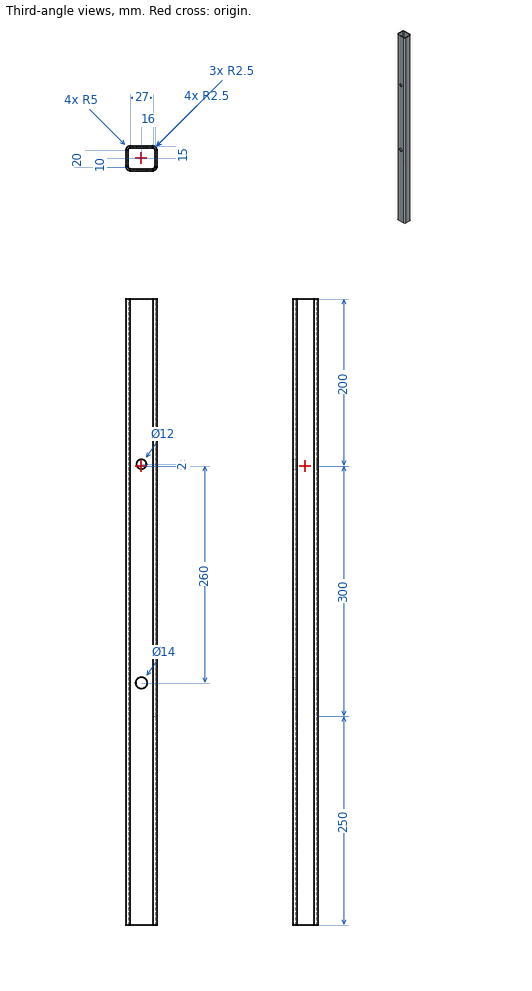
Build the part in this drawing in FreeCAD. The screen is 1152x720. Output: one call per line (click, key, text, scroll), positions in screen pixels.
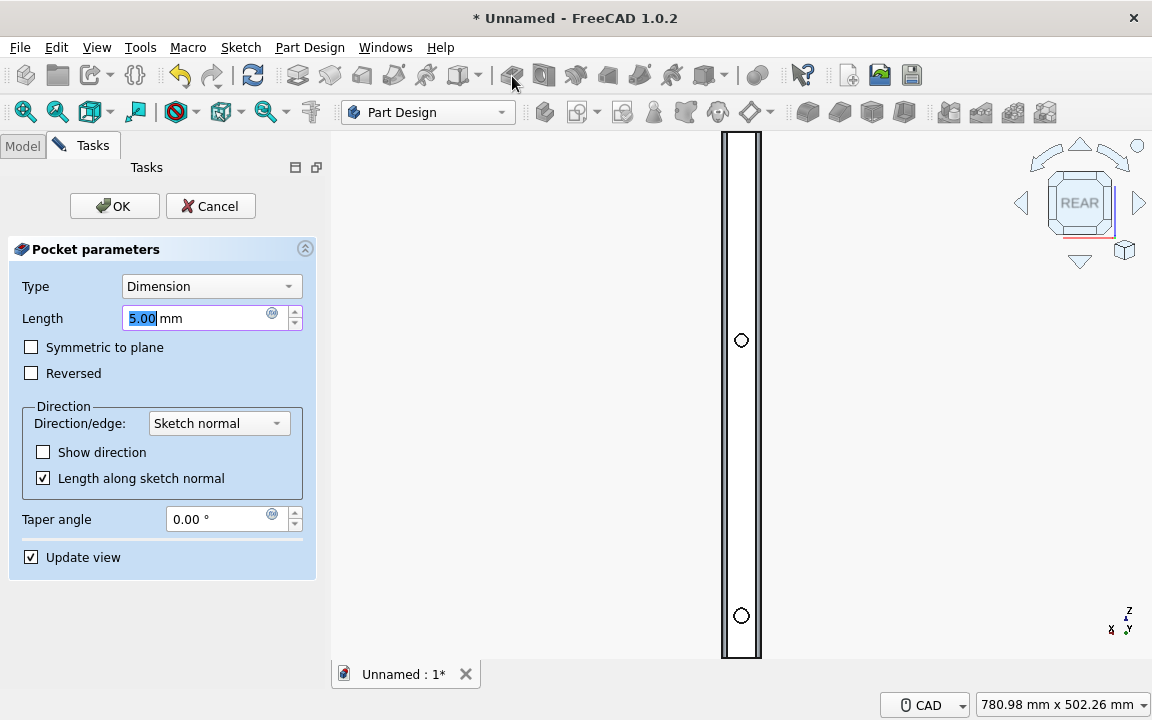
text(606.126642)
key(Tab)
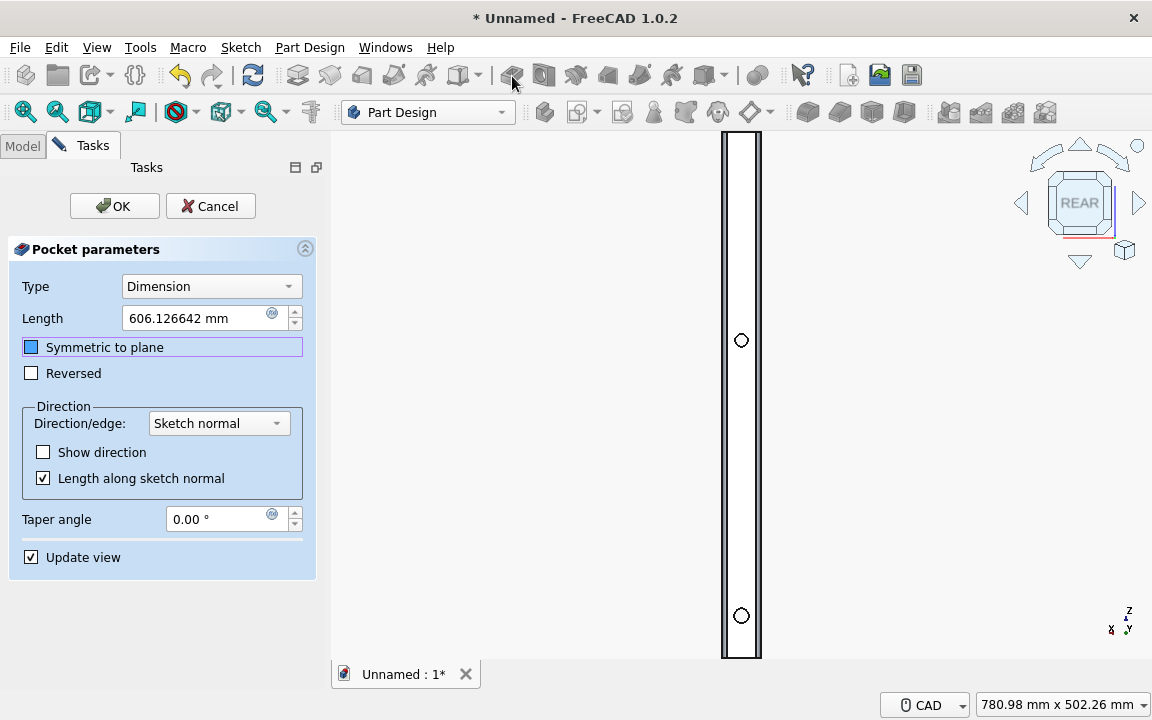
click(30, 347)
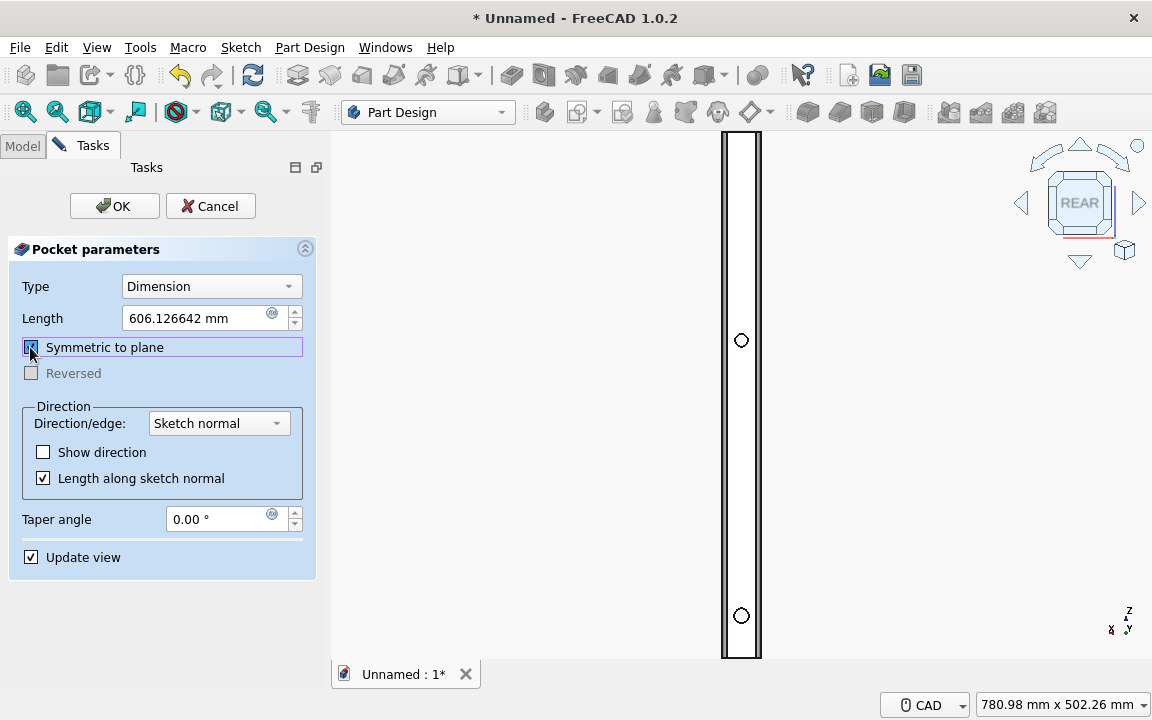
click(115, 206)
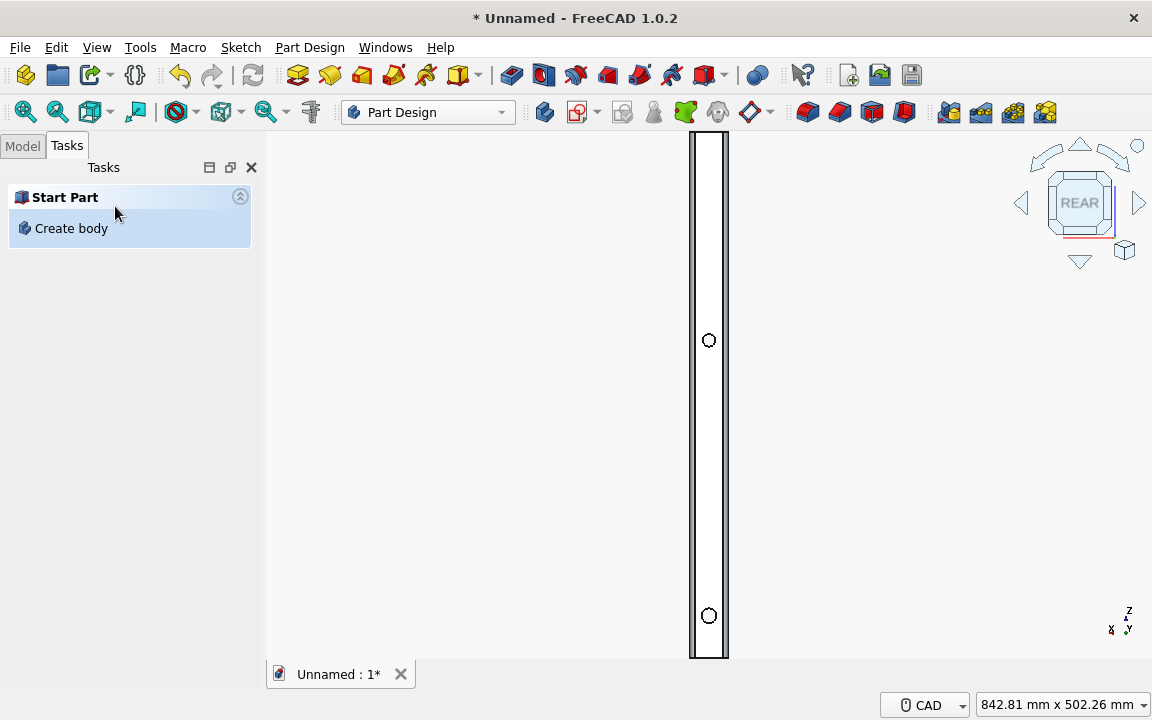
click(23, 145)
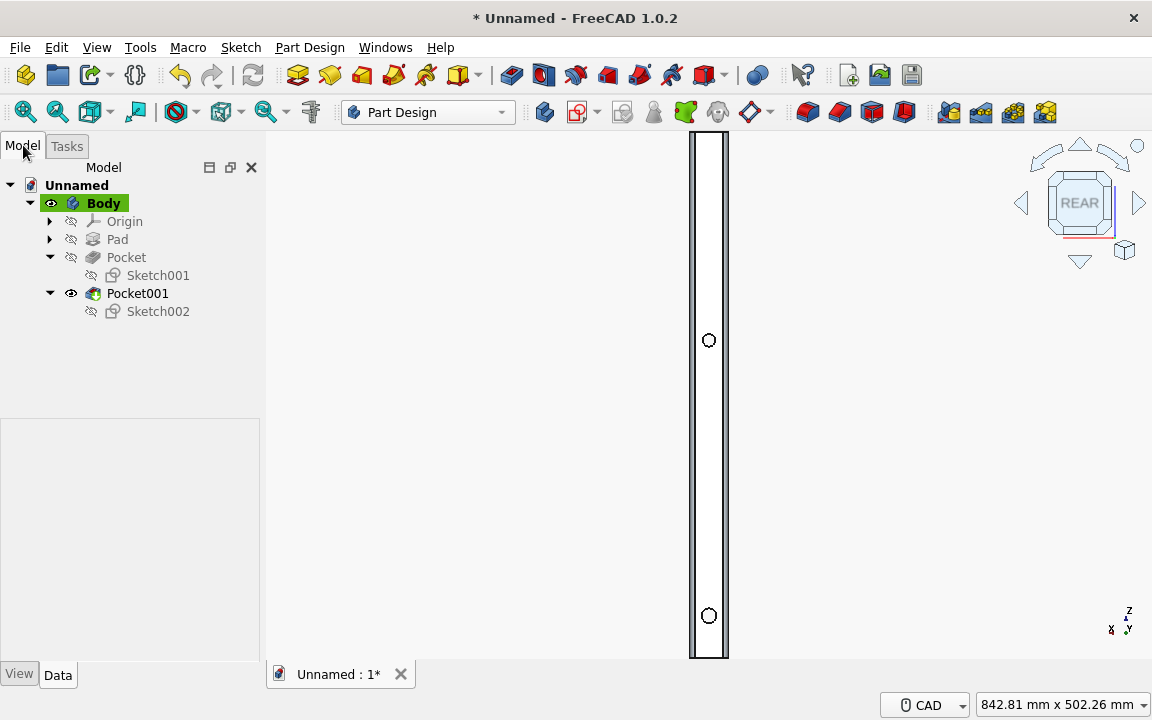
click(50, 221)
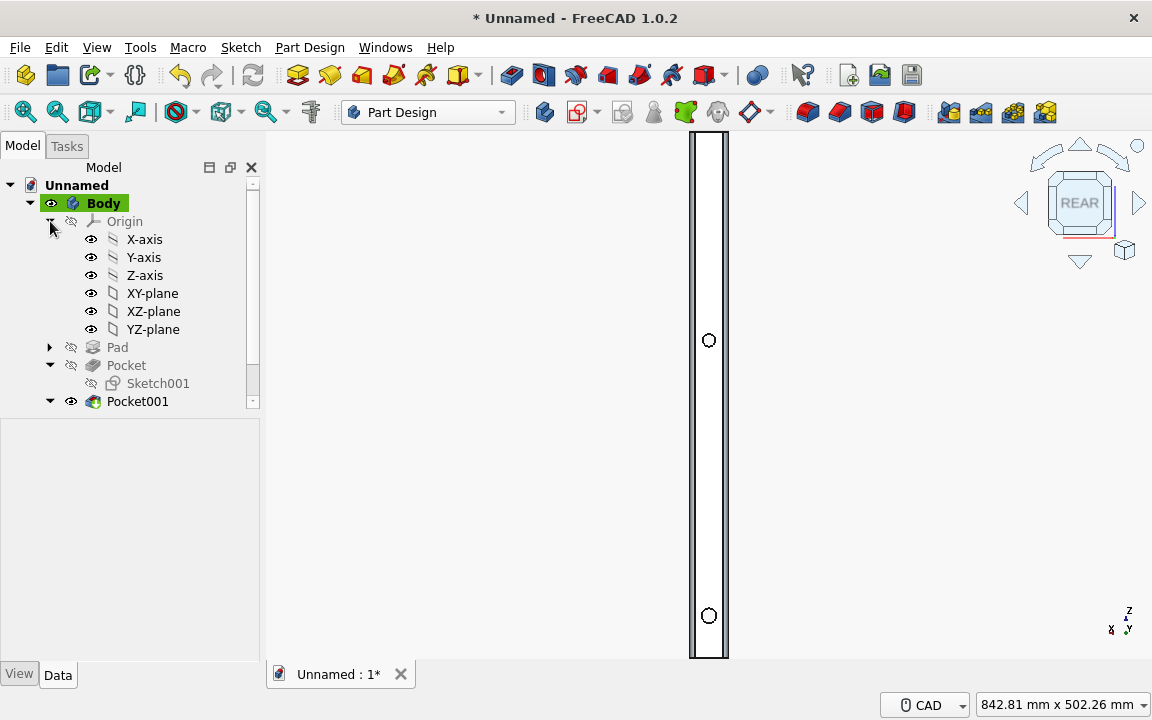
click(136, 293)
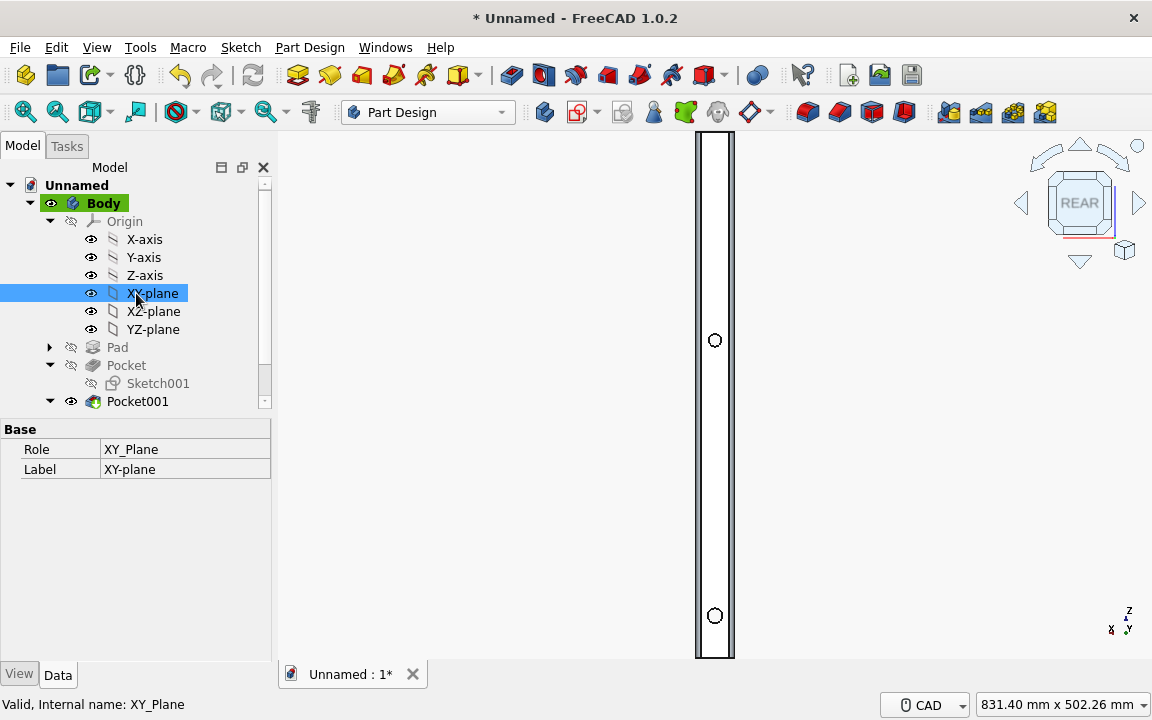
click(750, 112)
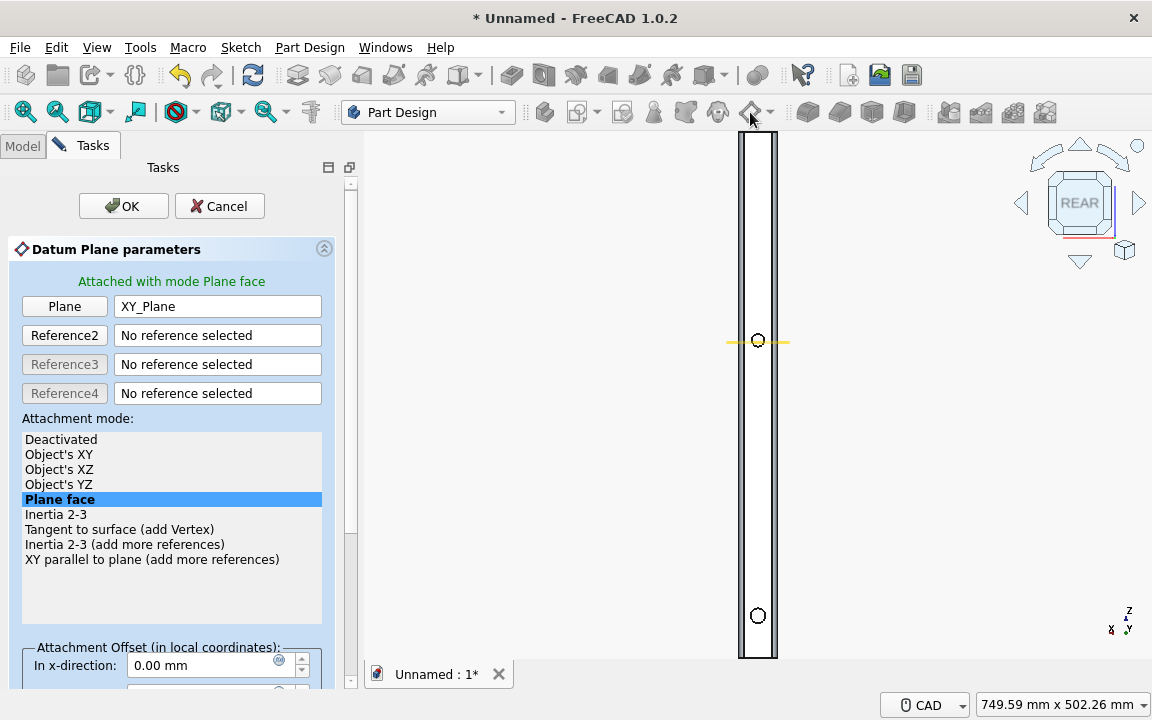
scroll(351, 432, down, 2)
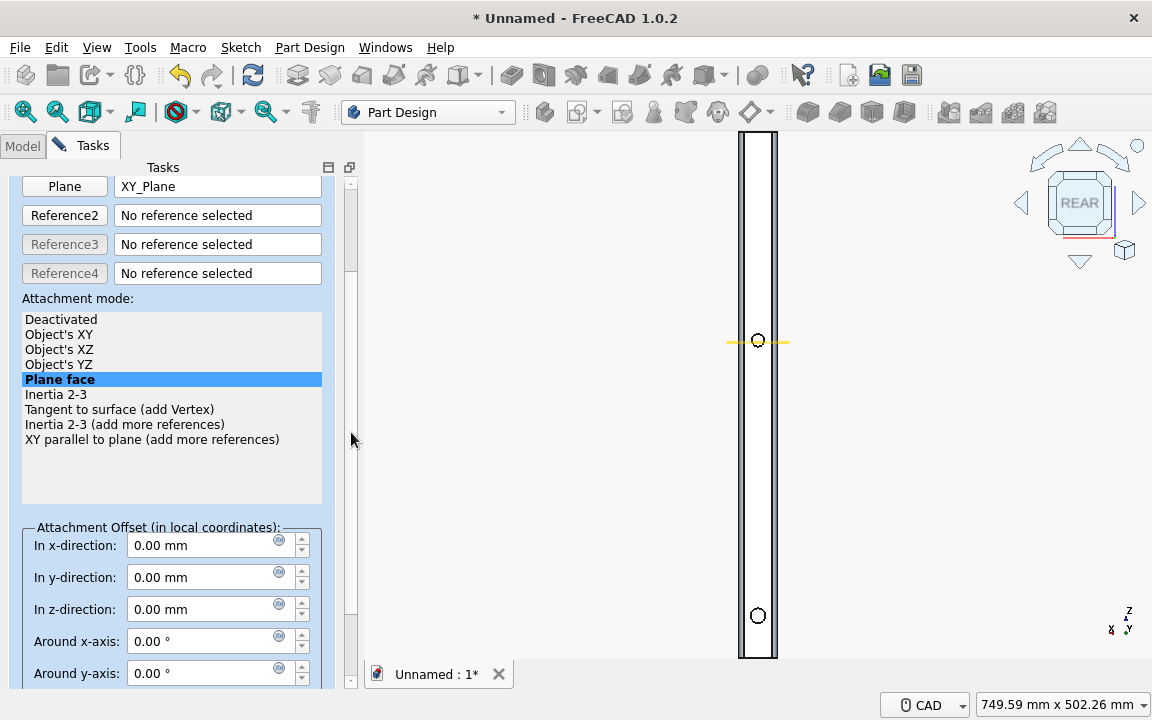
triple_click(210, 609)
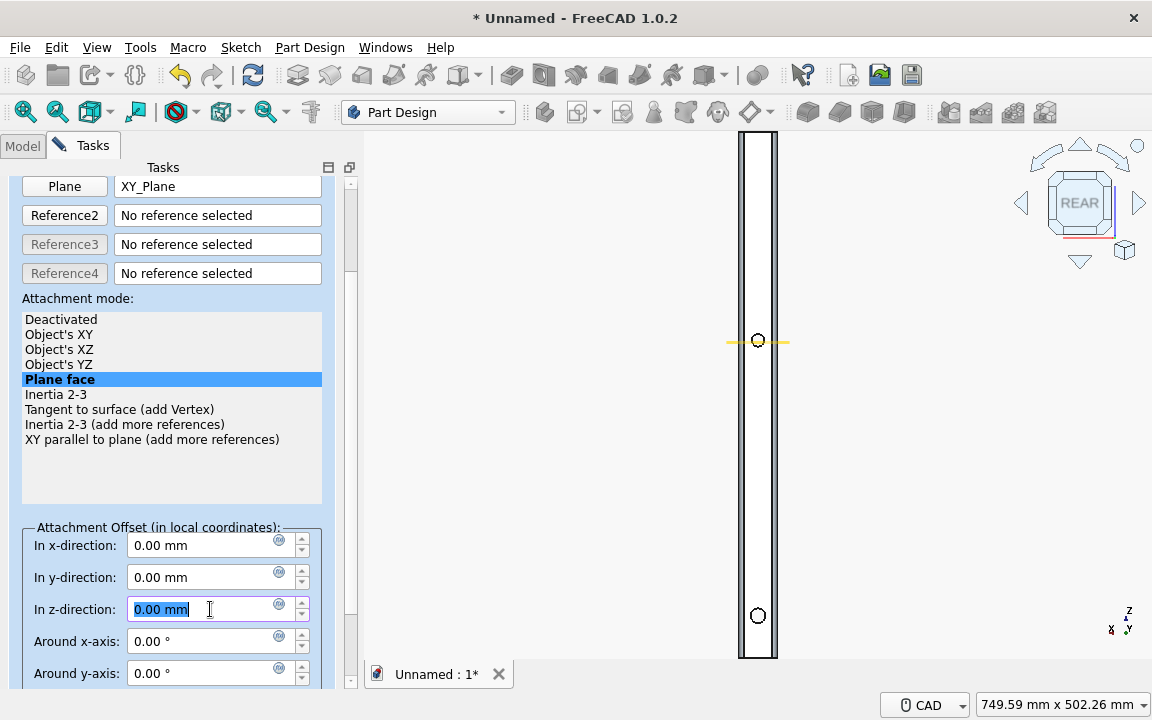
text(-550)
key(Tab)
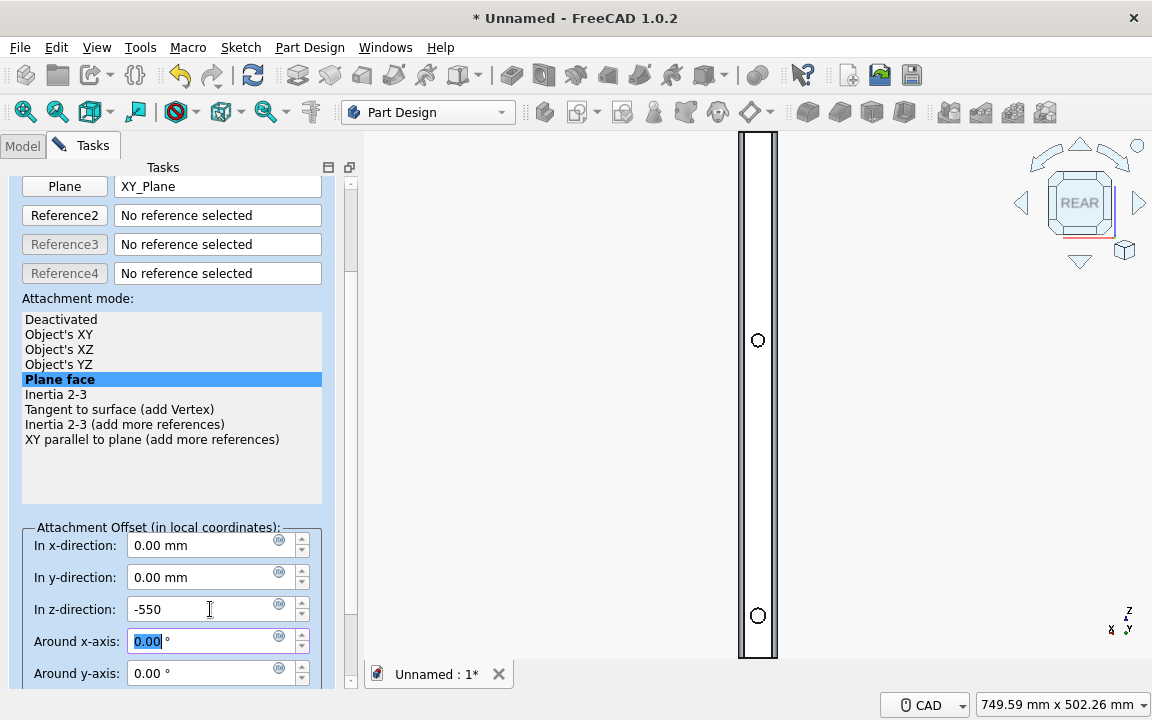
scroll(351, 432, up, 3)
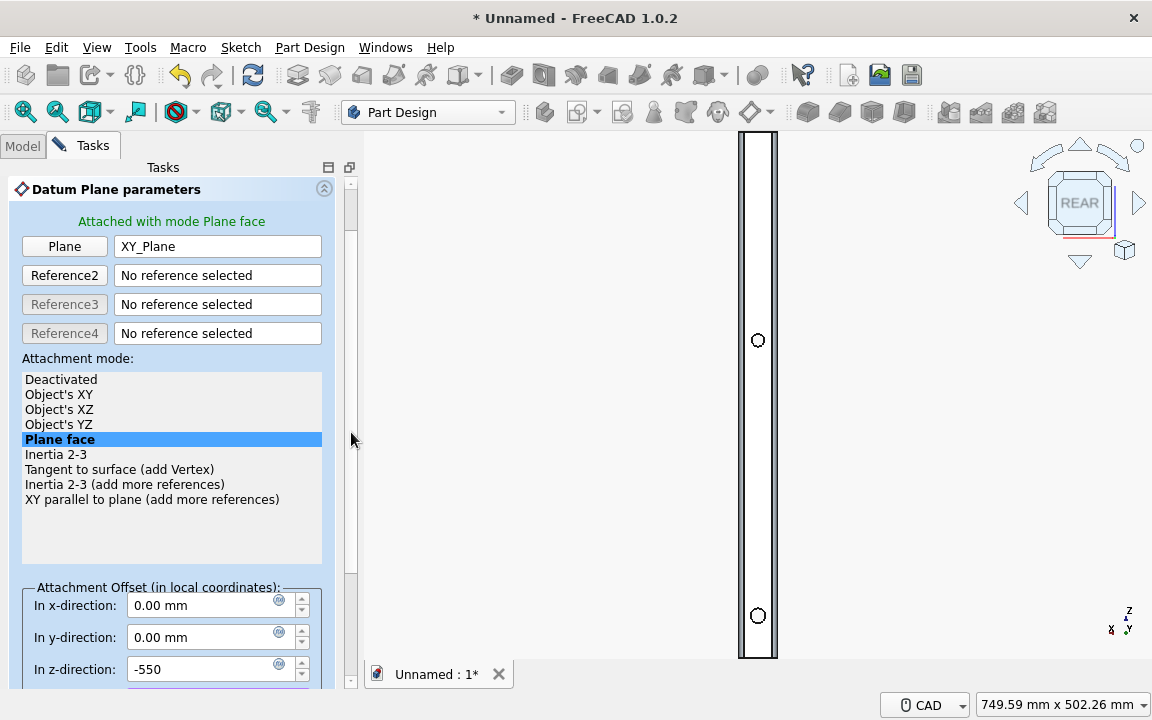
click(124, 206)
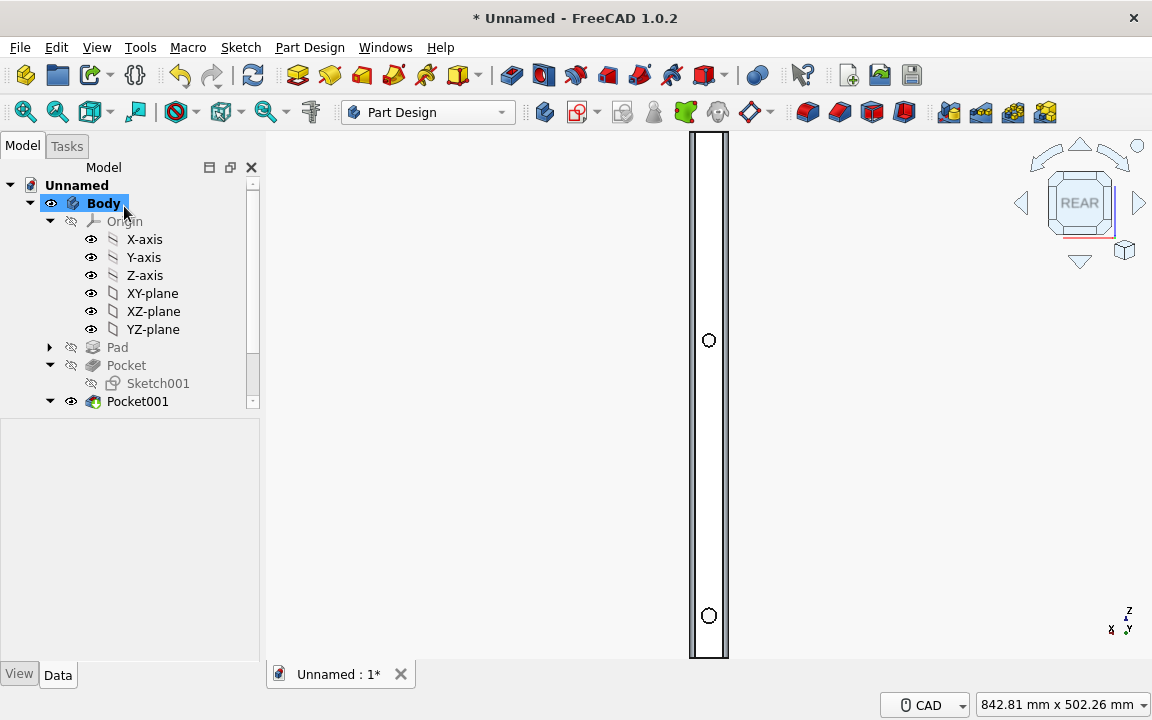
scroll(100, 289, down, 3)